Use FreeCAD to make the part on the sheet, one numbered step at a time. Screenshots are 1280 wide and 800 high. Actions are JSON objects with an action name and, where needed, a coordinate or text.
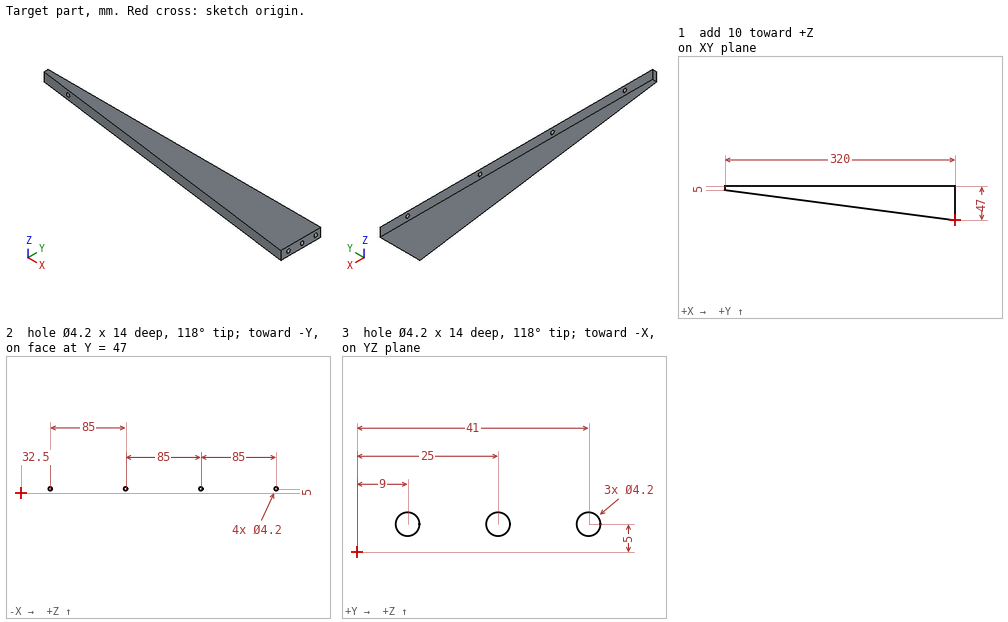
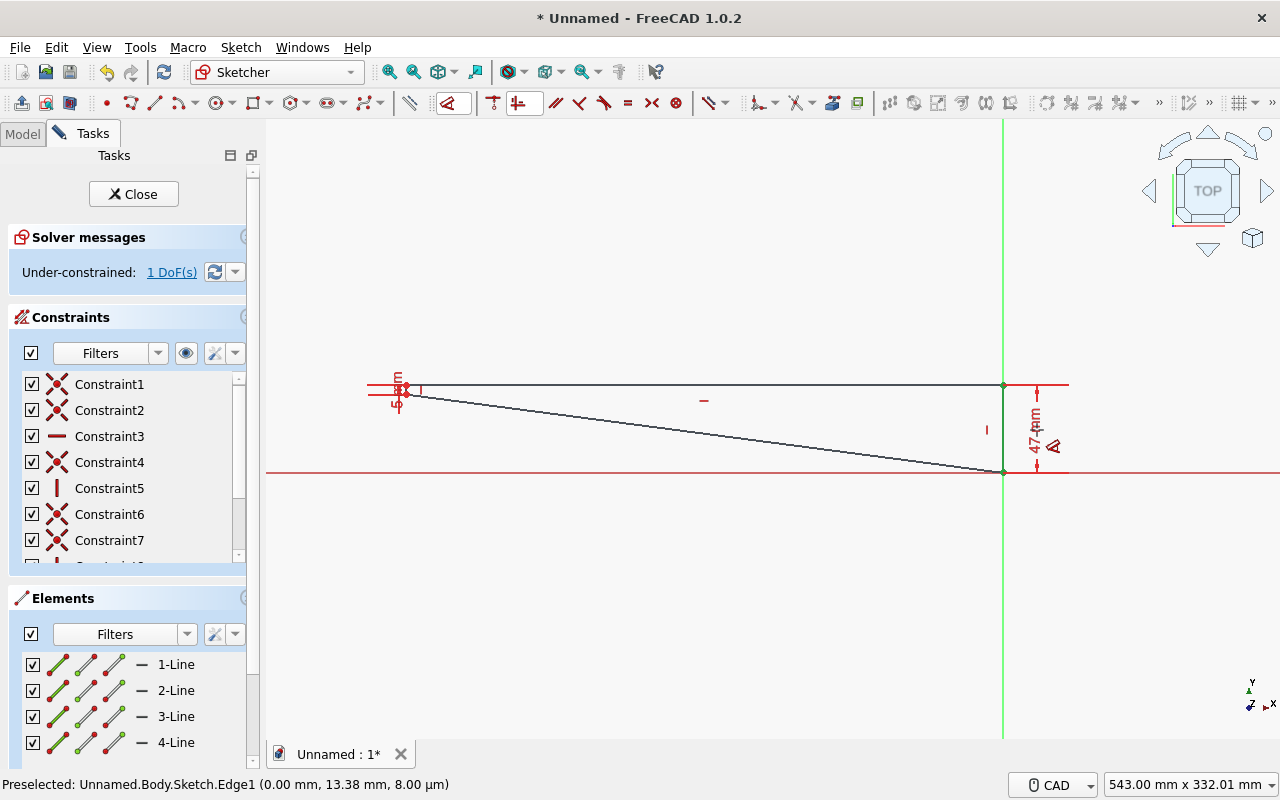
{"action": "left_click", "coordinate": [824, 385]}
{"action": "left_click", "coordinate": [705, 351]}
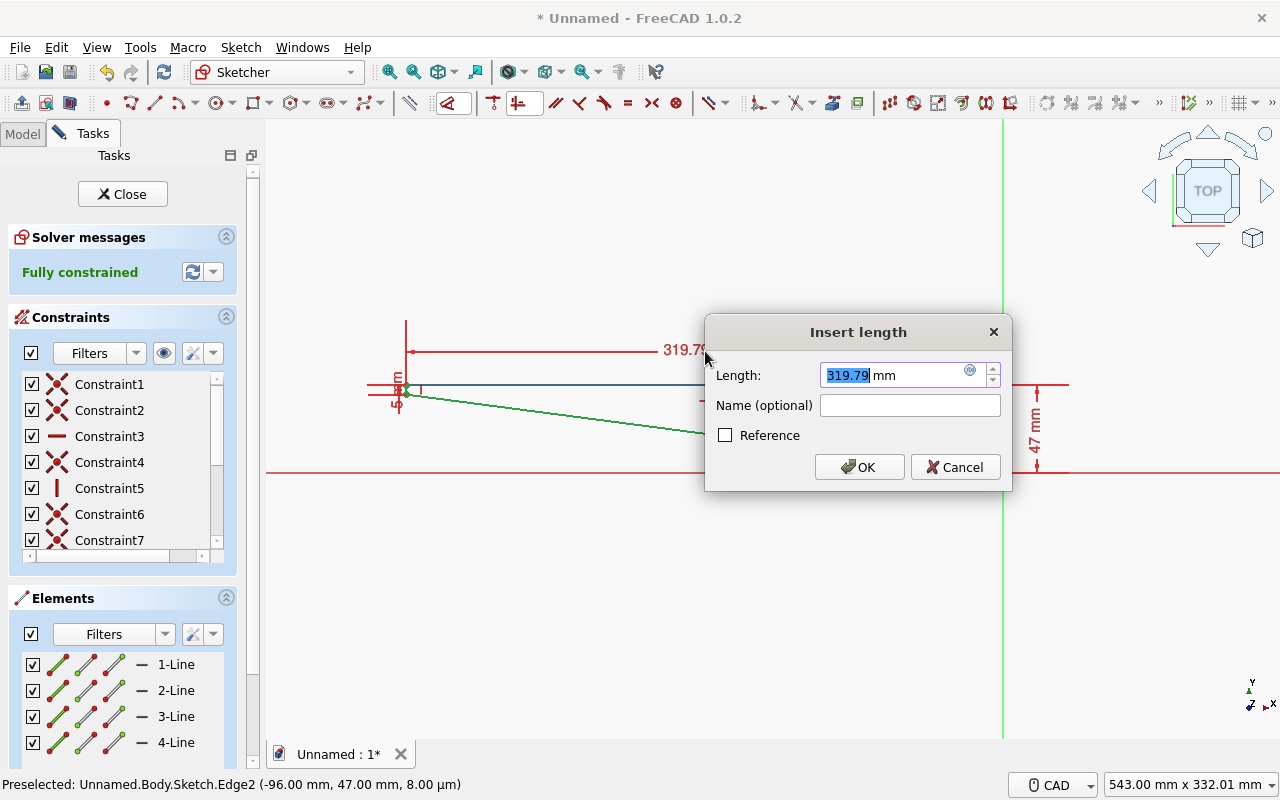
{"action": "type", "text": "320"}
{"action": "key", "text": "Return"}
{"action": "key", "text": "Escape"}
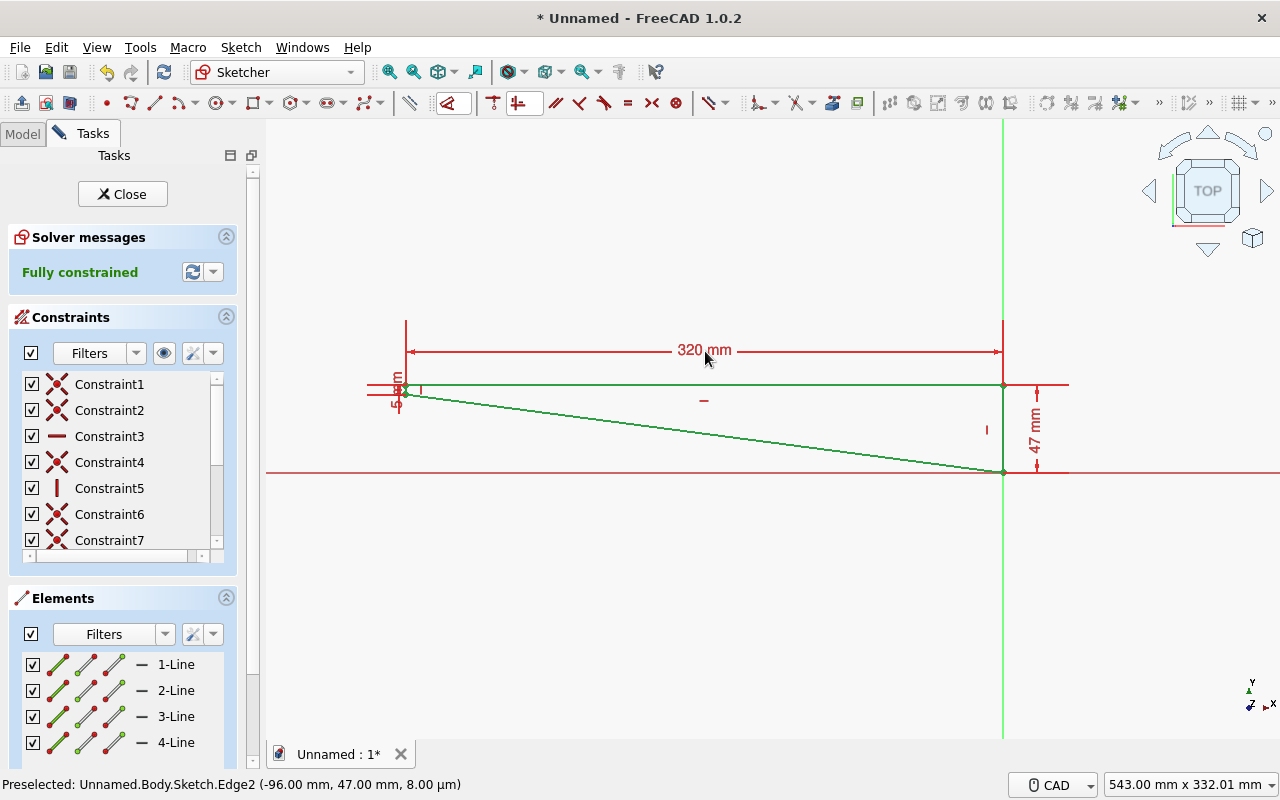
{"action": "left_click", "coordinate": [123, 194]}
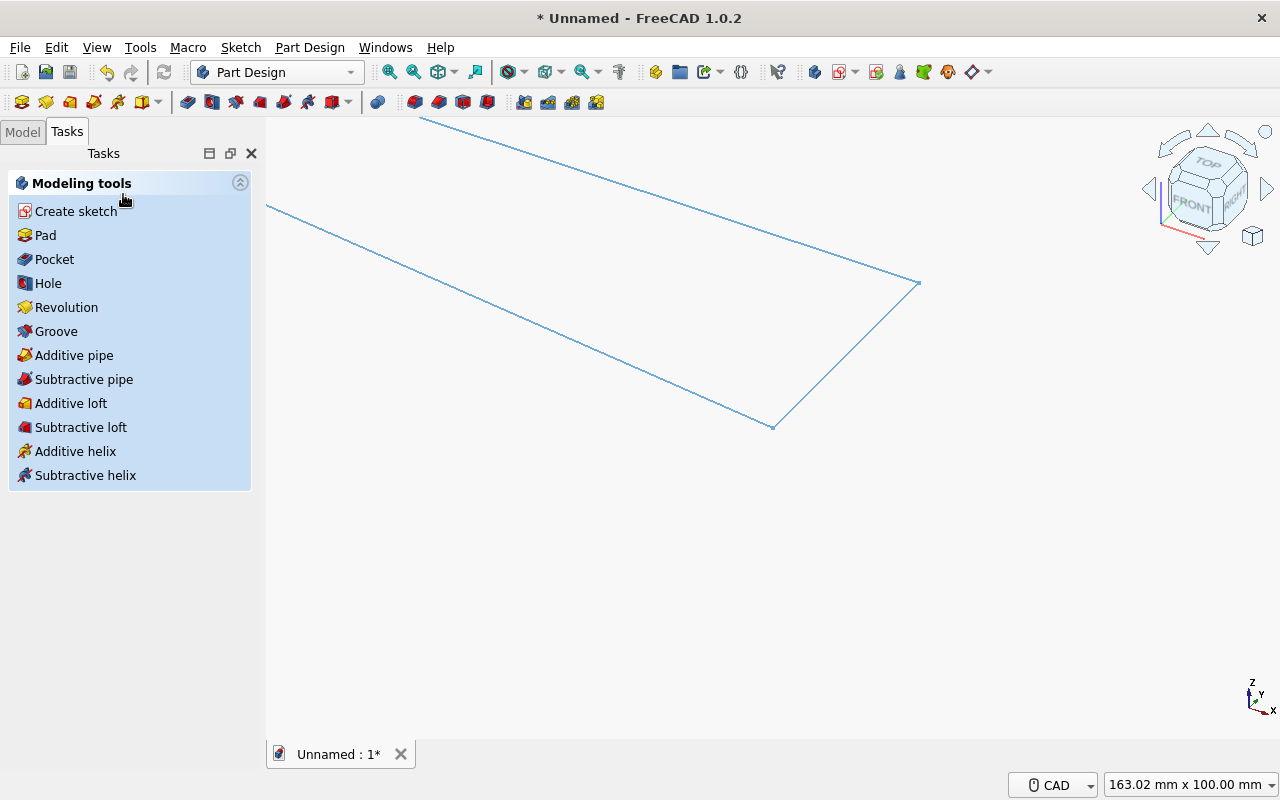
{"action": "left_click", "coordinate": [22, 102]}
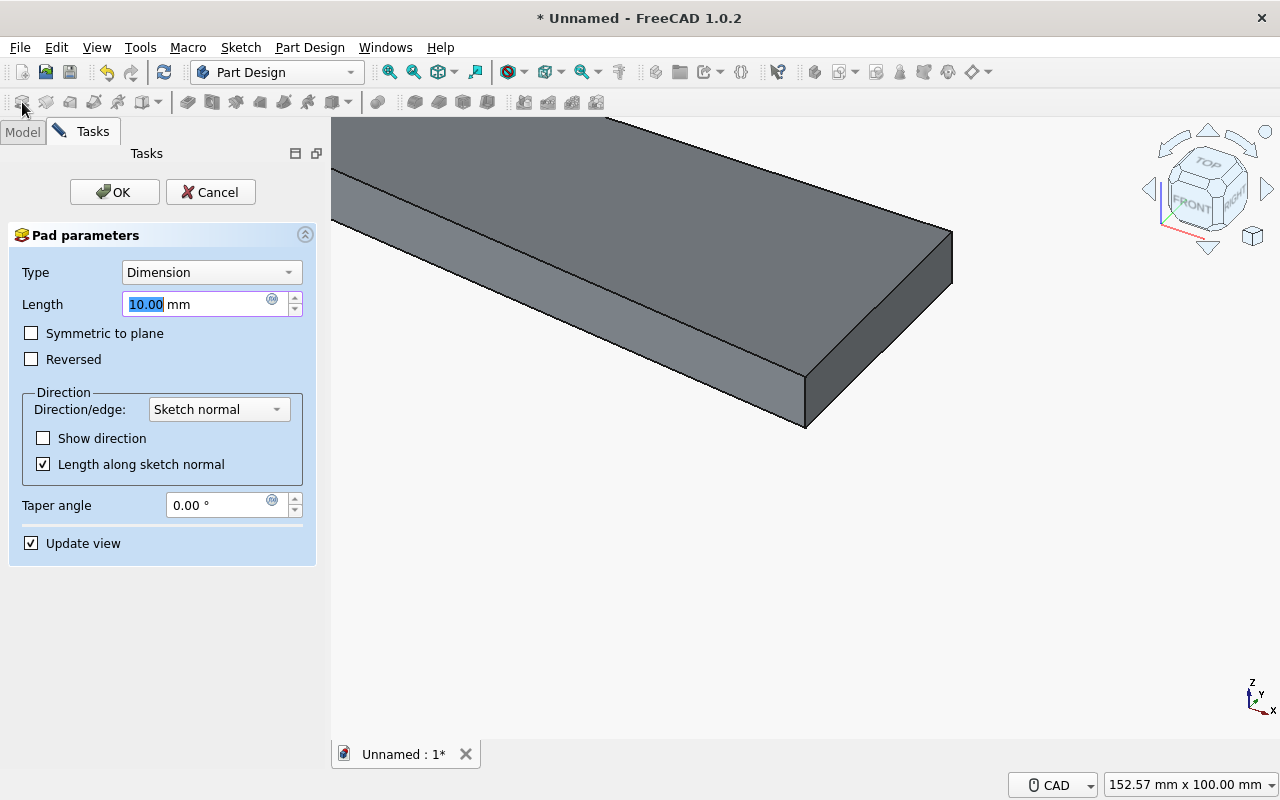
{"action": "type", "text": "10"}
{"action": "key", "text": "Tab"}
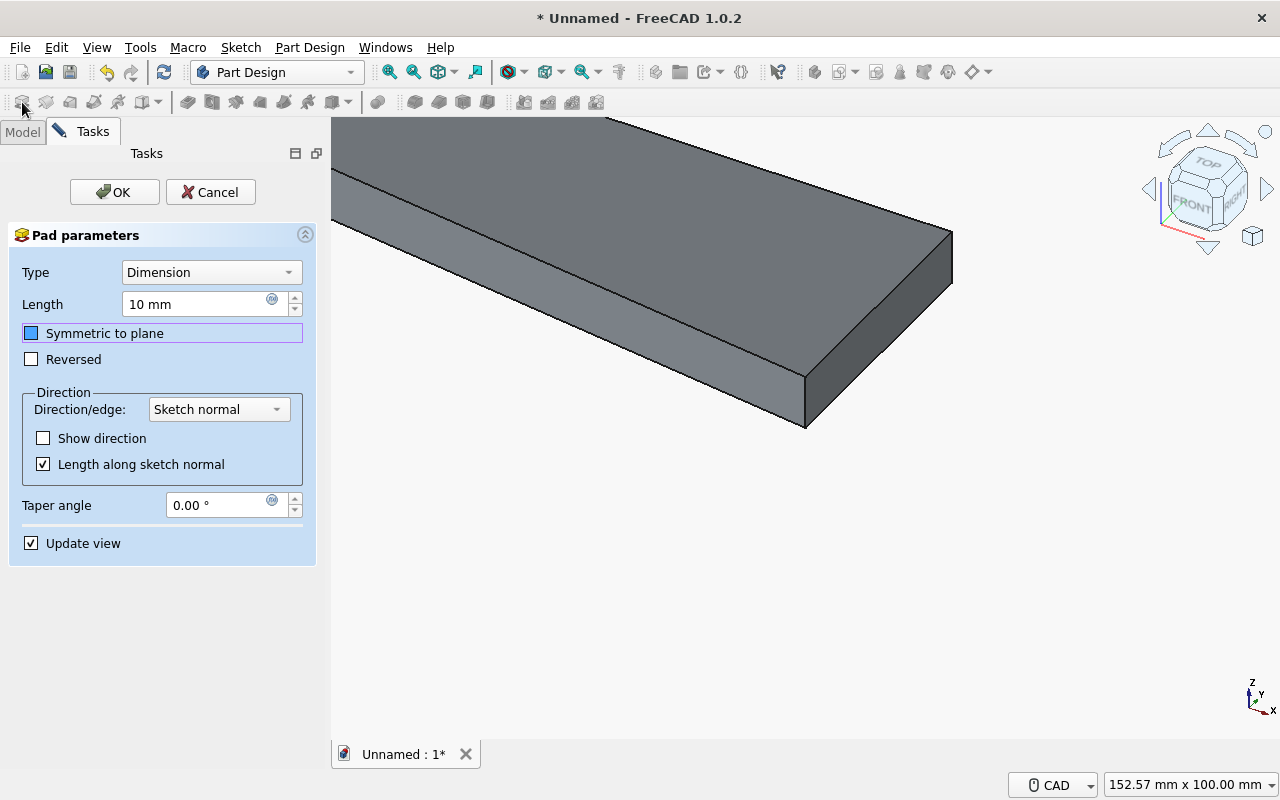
{"action": "left_click", "coordinate": [115, 192]}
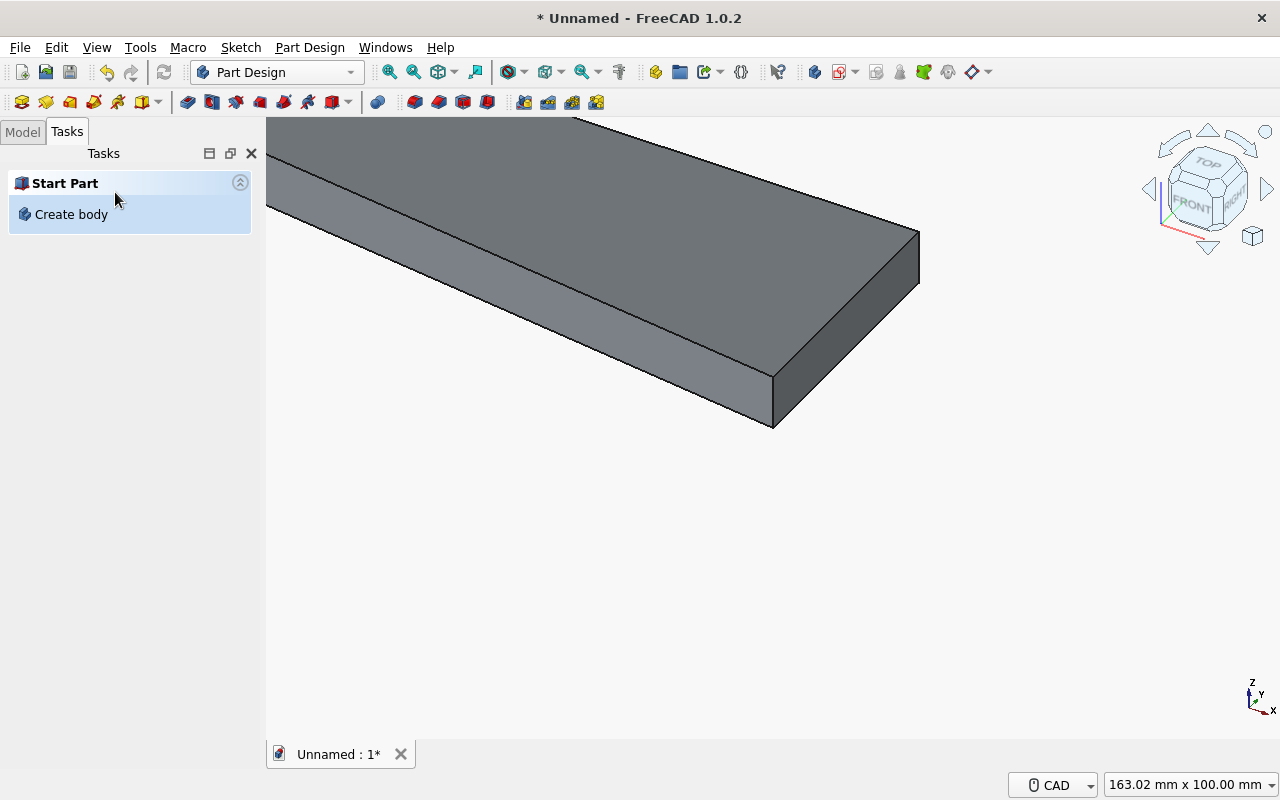
{"action": "left_click", "coordinate": [390, 72]}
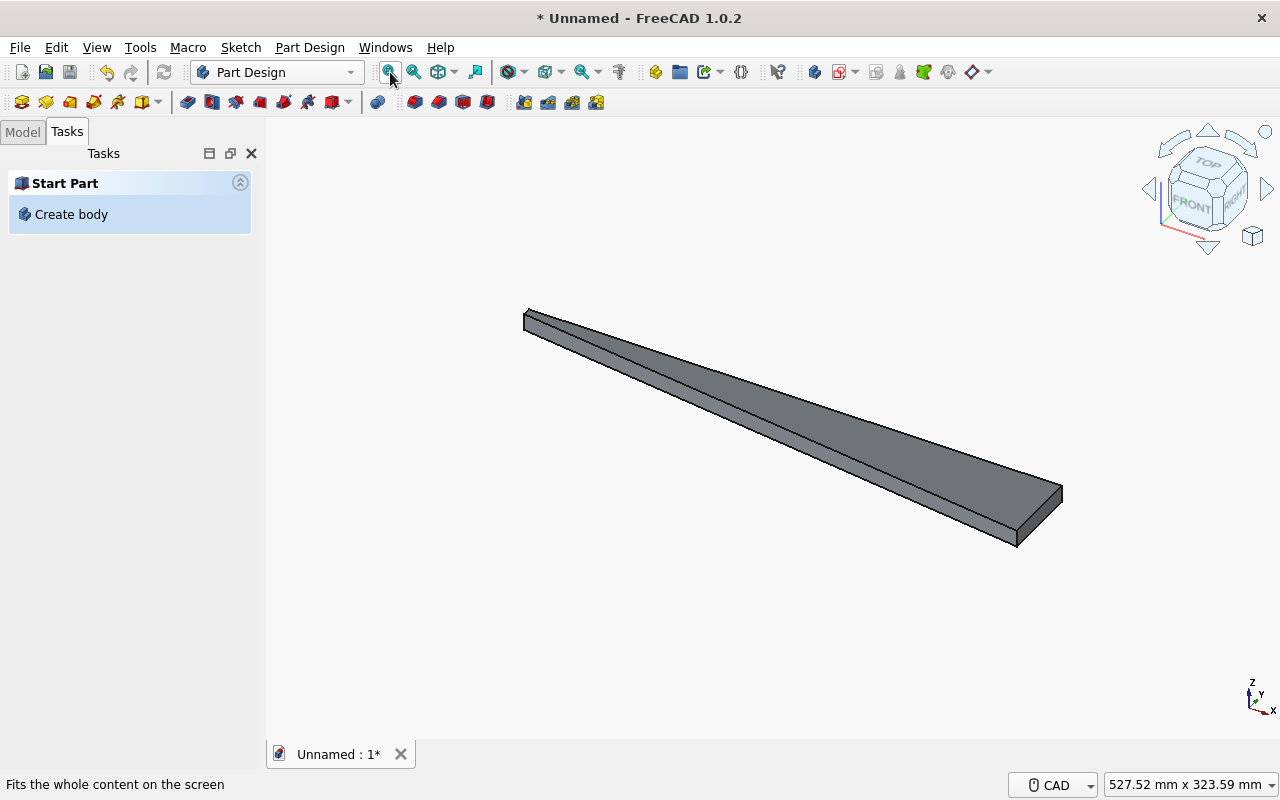
{"action": "key", "text": "4"}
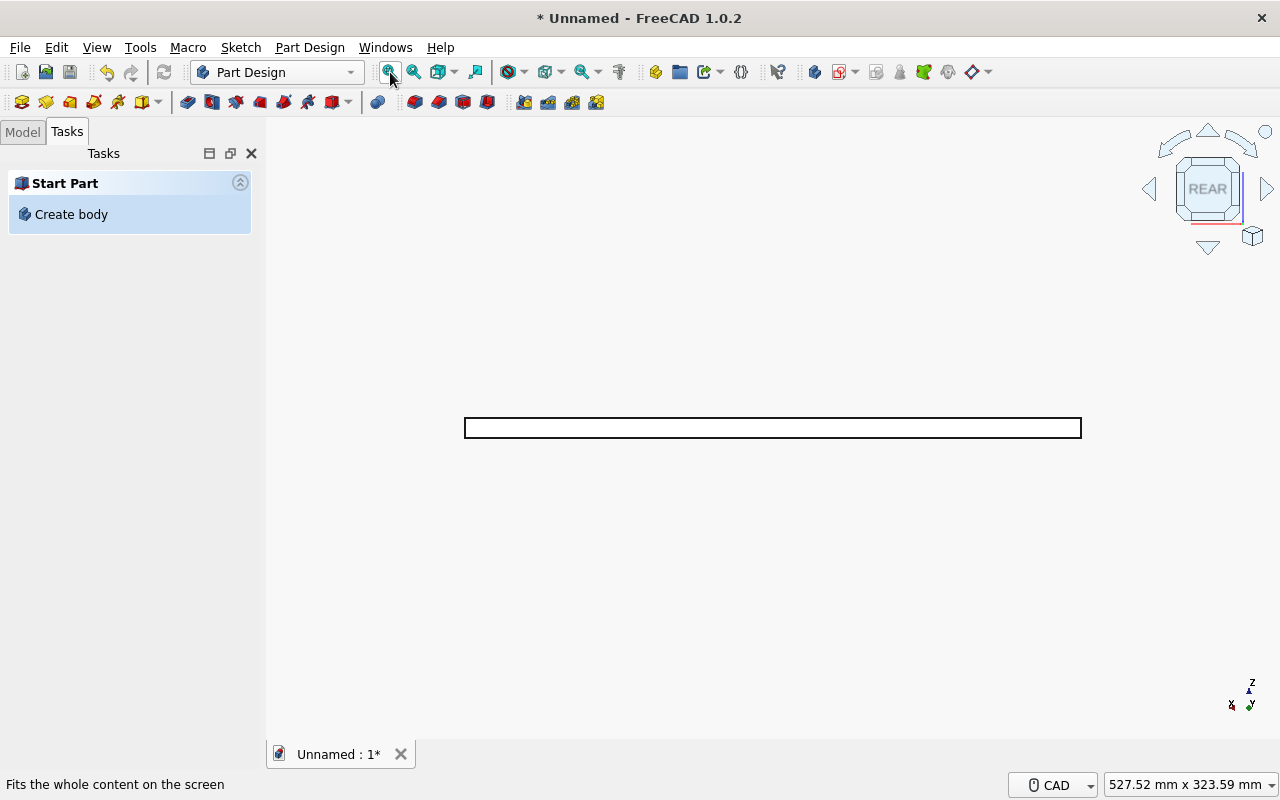
{"action": "left_click", "coordinate": [509, 427]}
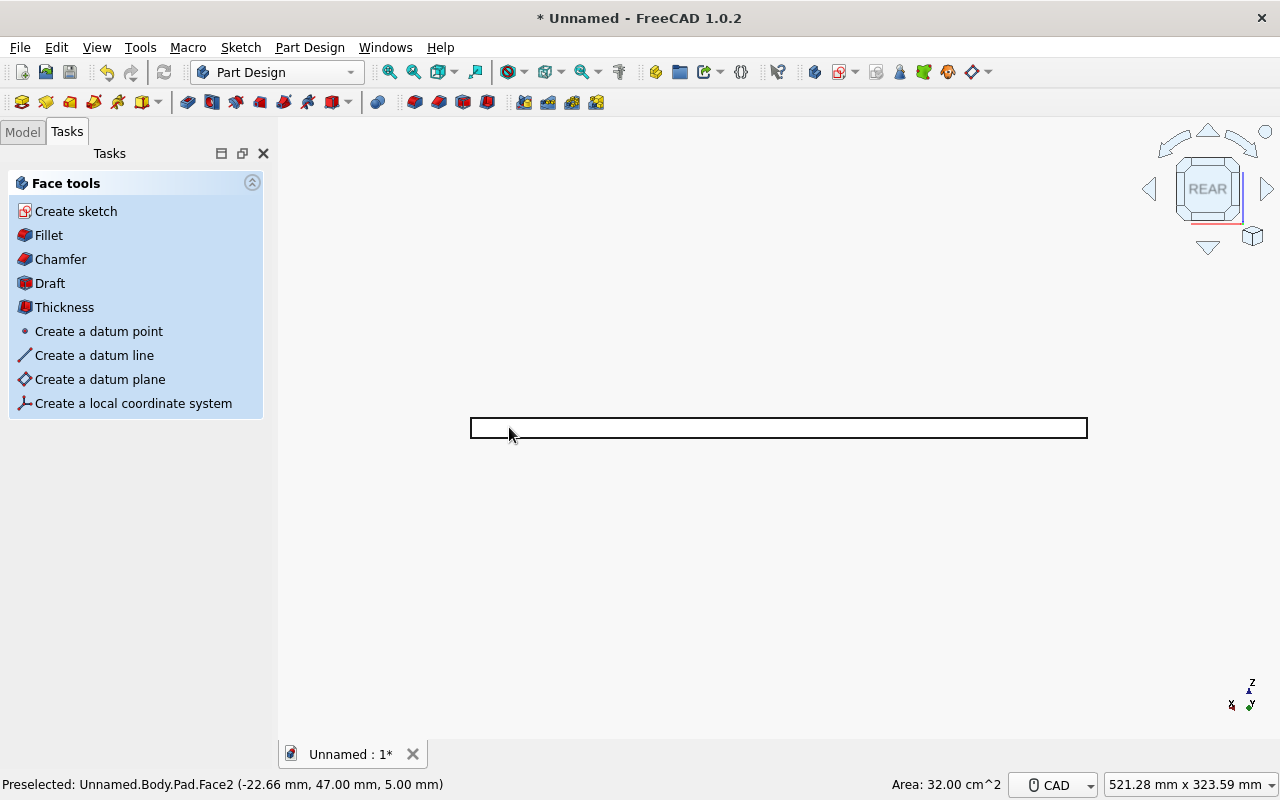
{"action": "left_click", "coordinate": [840, 72]}